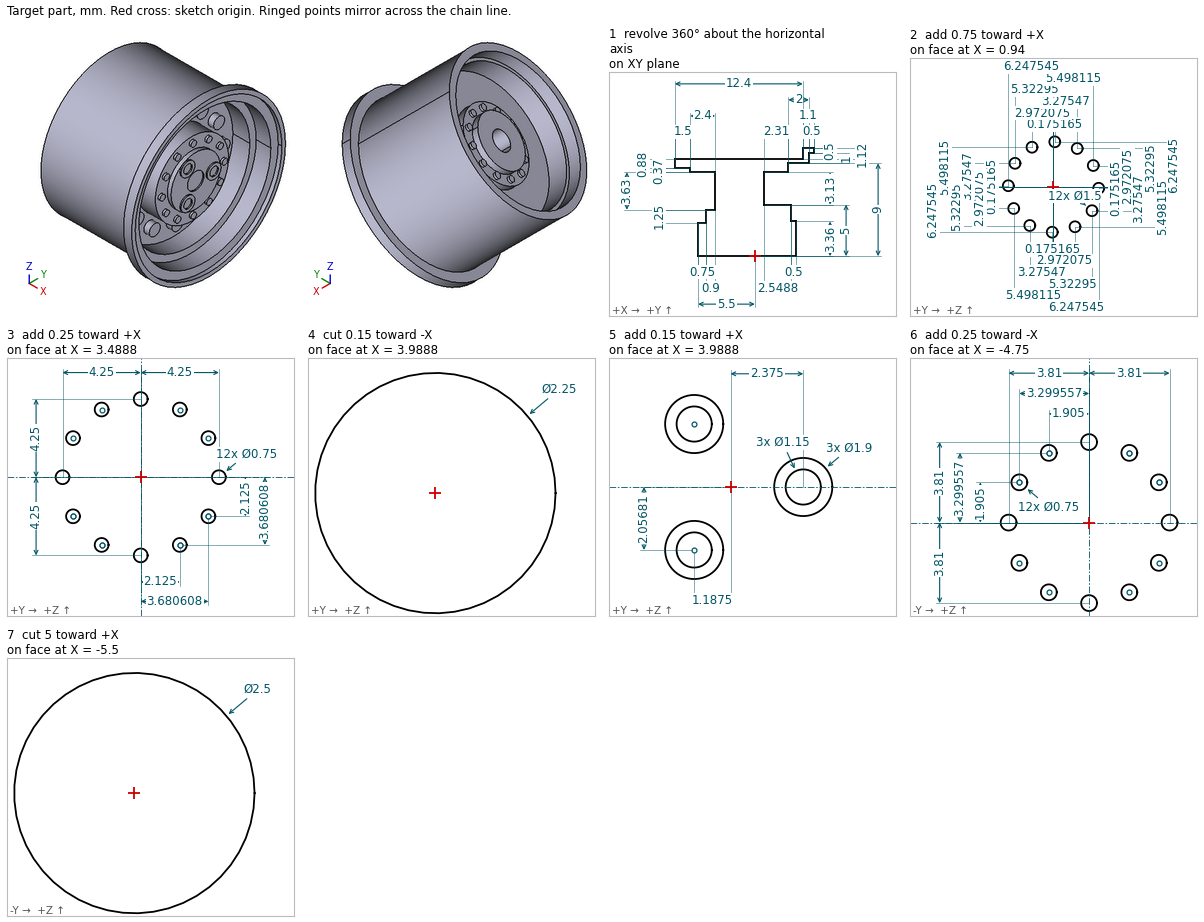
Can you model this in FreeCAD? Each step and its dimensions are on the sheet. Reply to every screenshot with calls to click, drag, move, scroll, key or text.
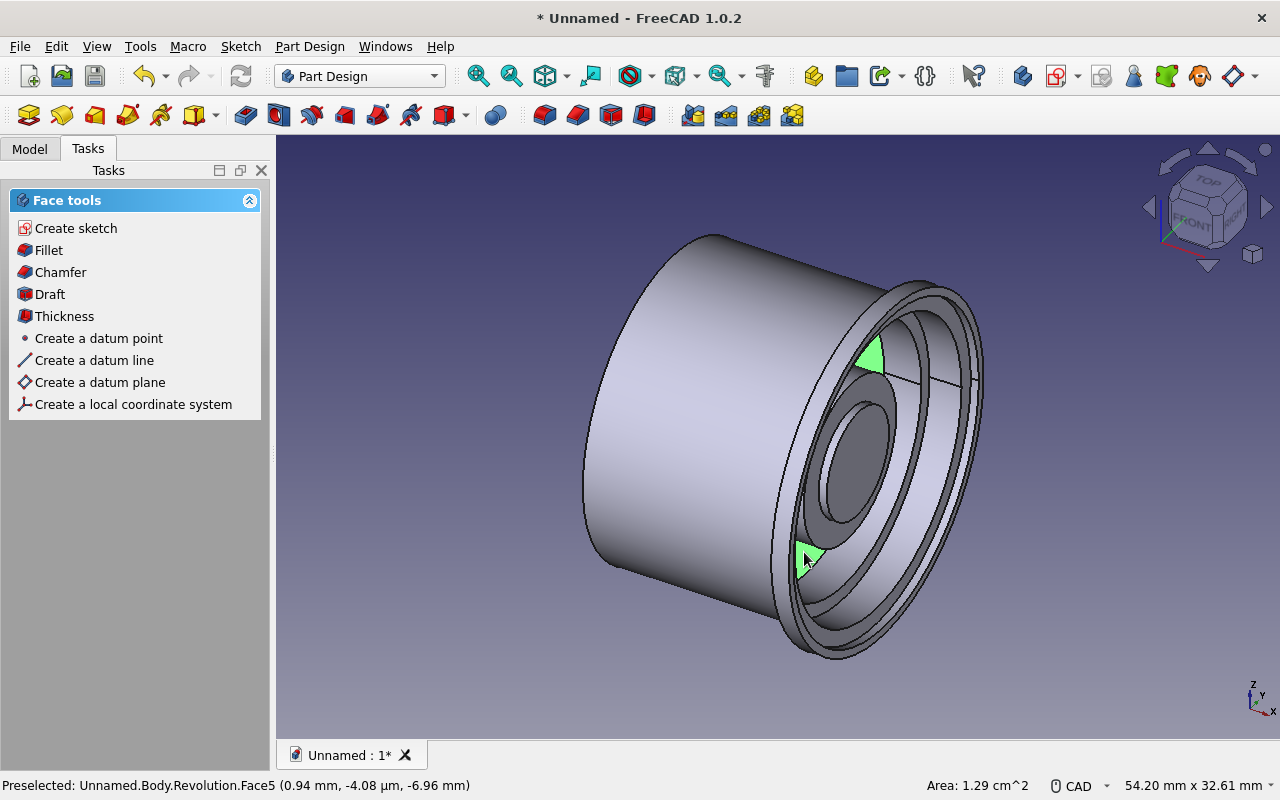
click(1056, 76)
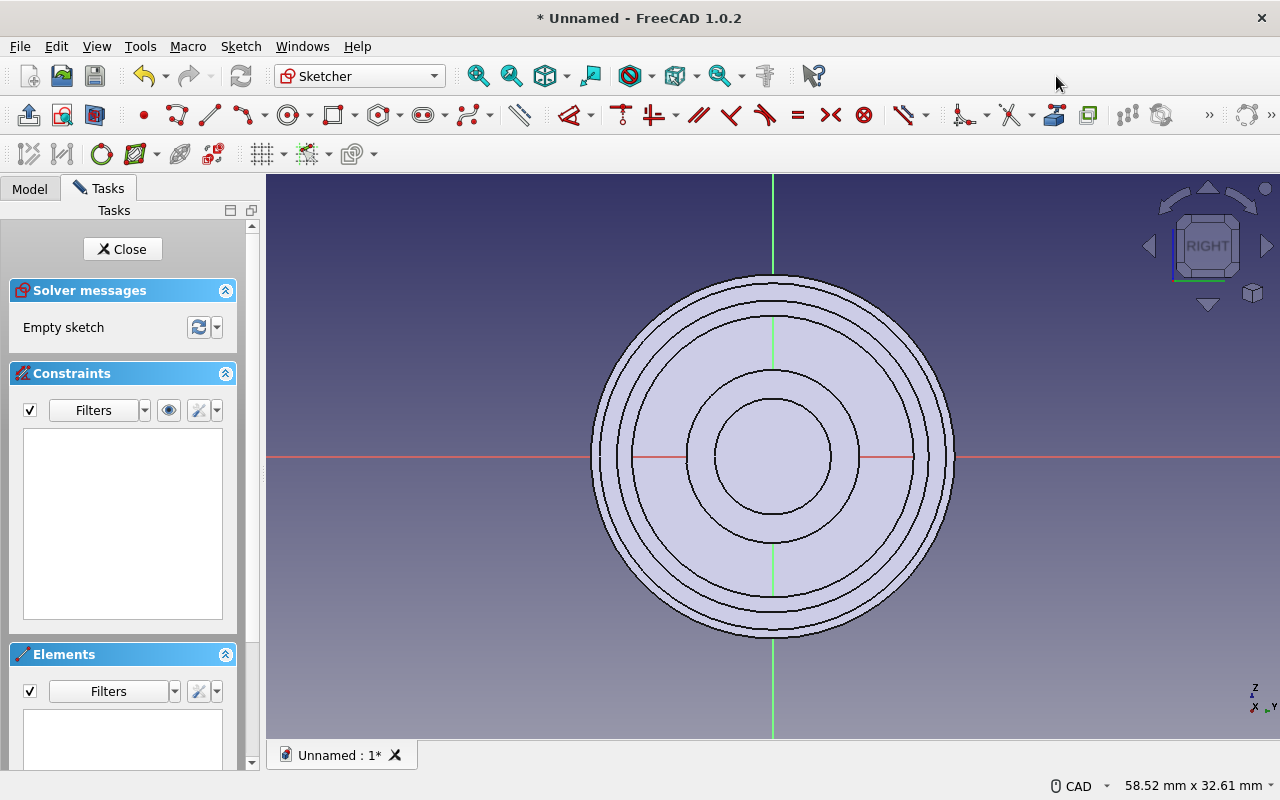
click(95, 116)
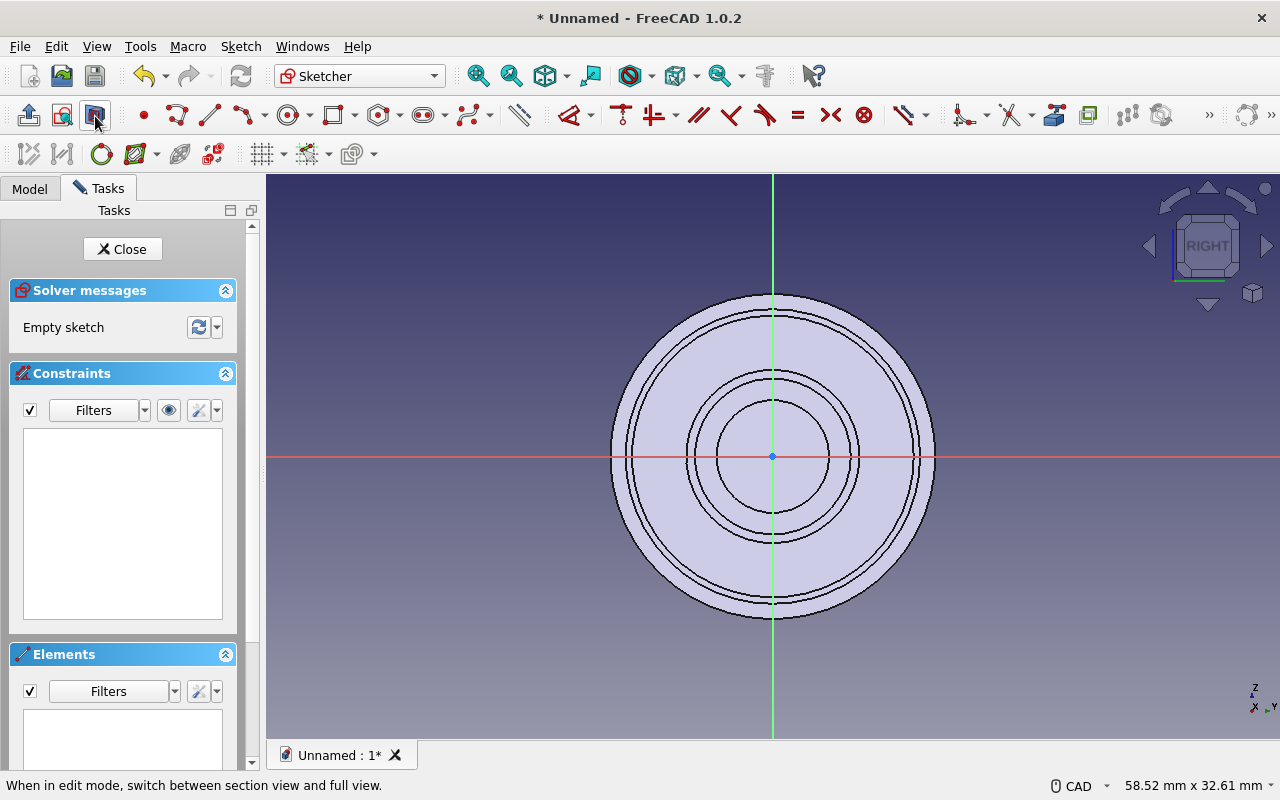
scroll(912, 456, up, 2)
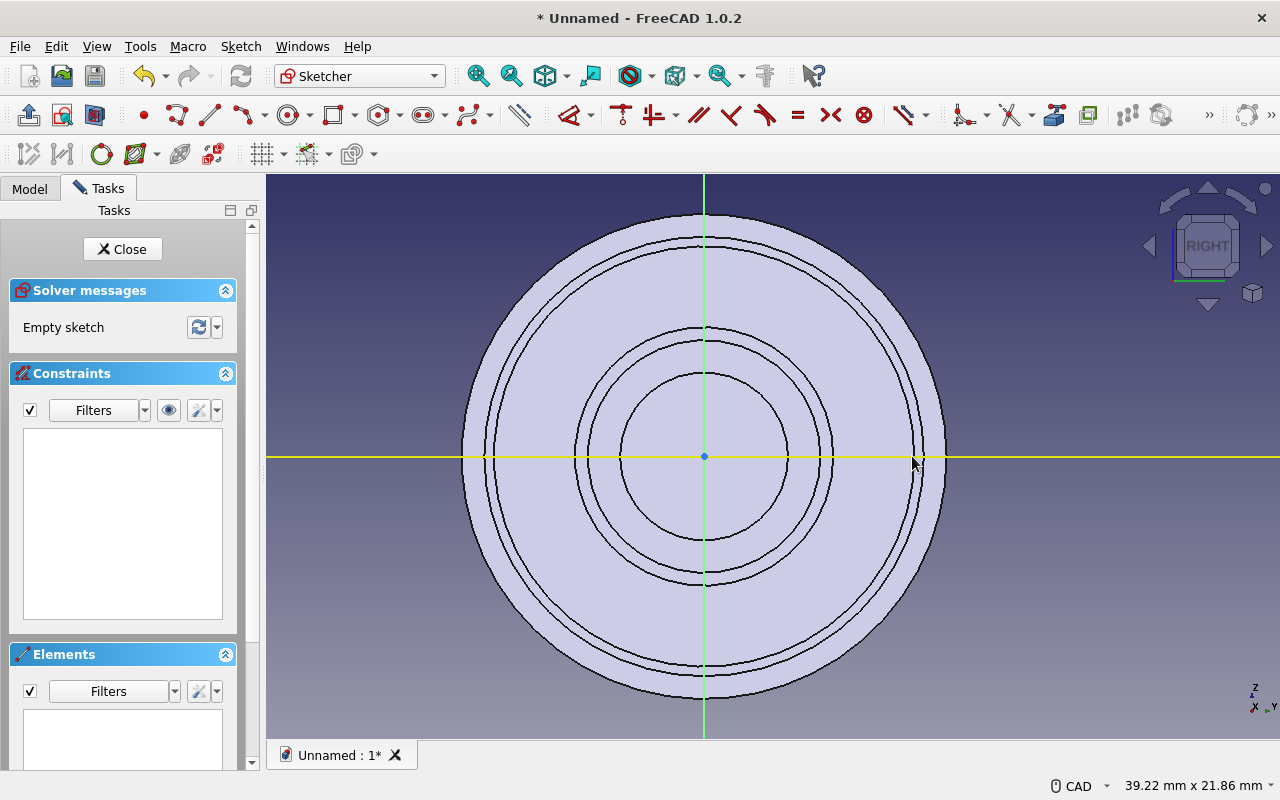
click(288, 116)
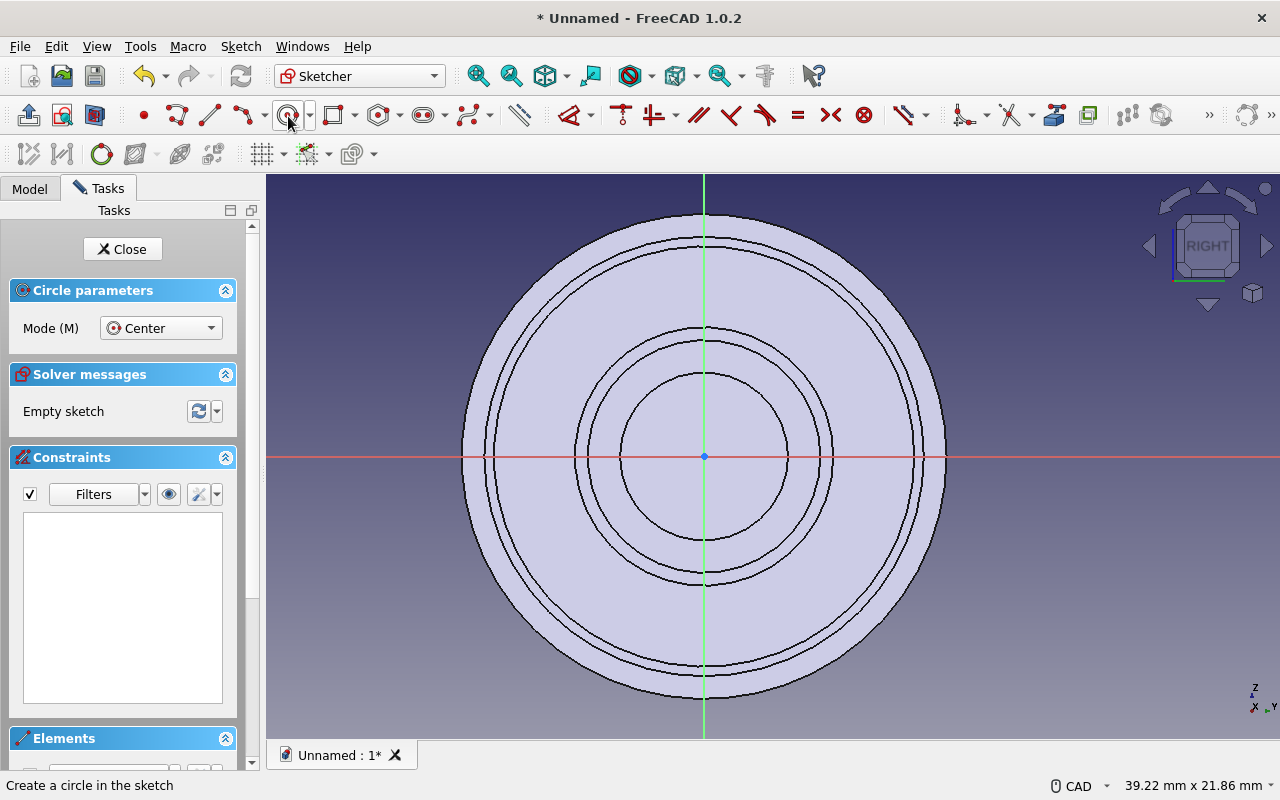
scroll(866, 461, up, 7)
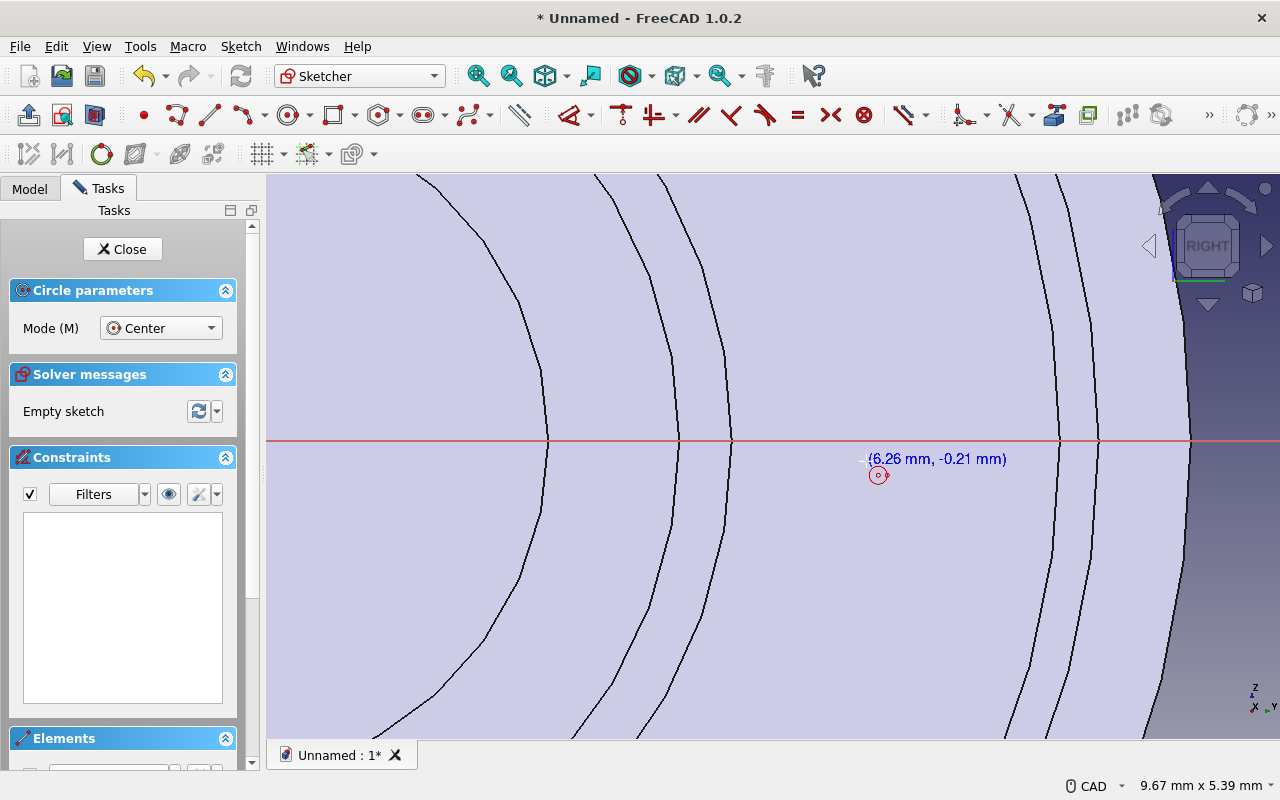
click(863, 460)
move(918, 404)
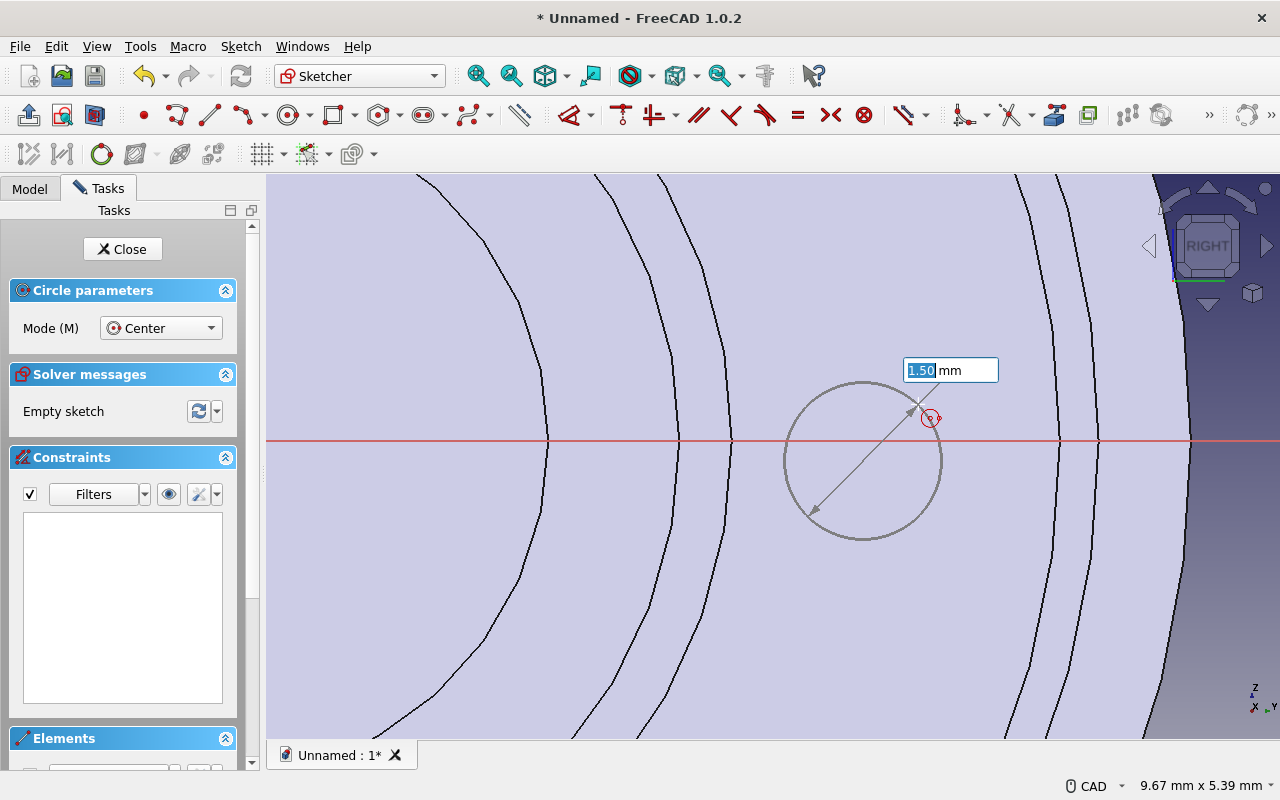
text(1.5)
key(Return)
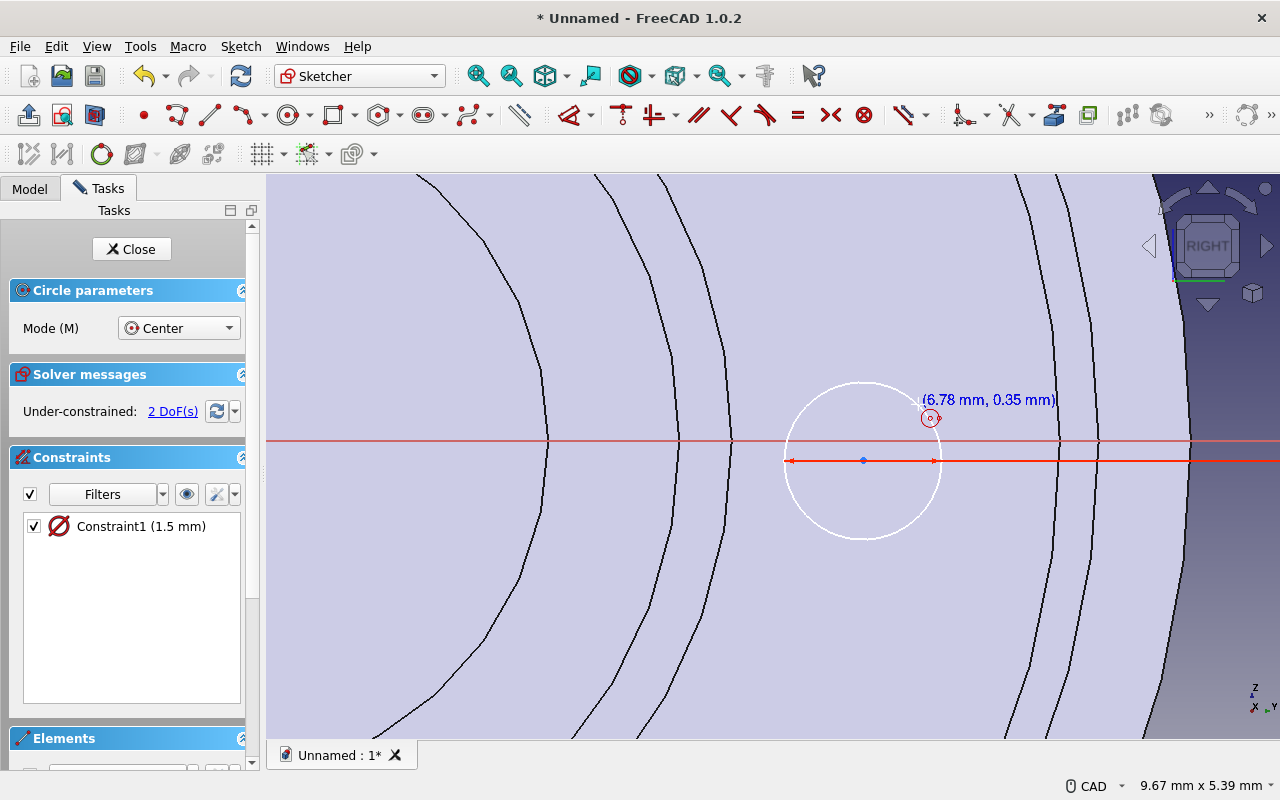
scroll(867, 462, down, 7)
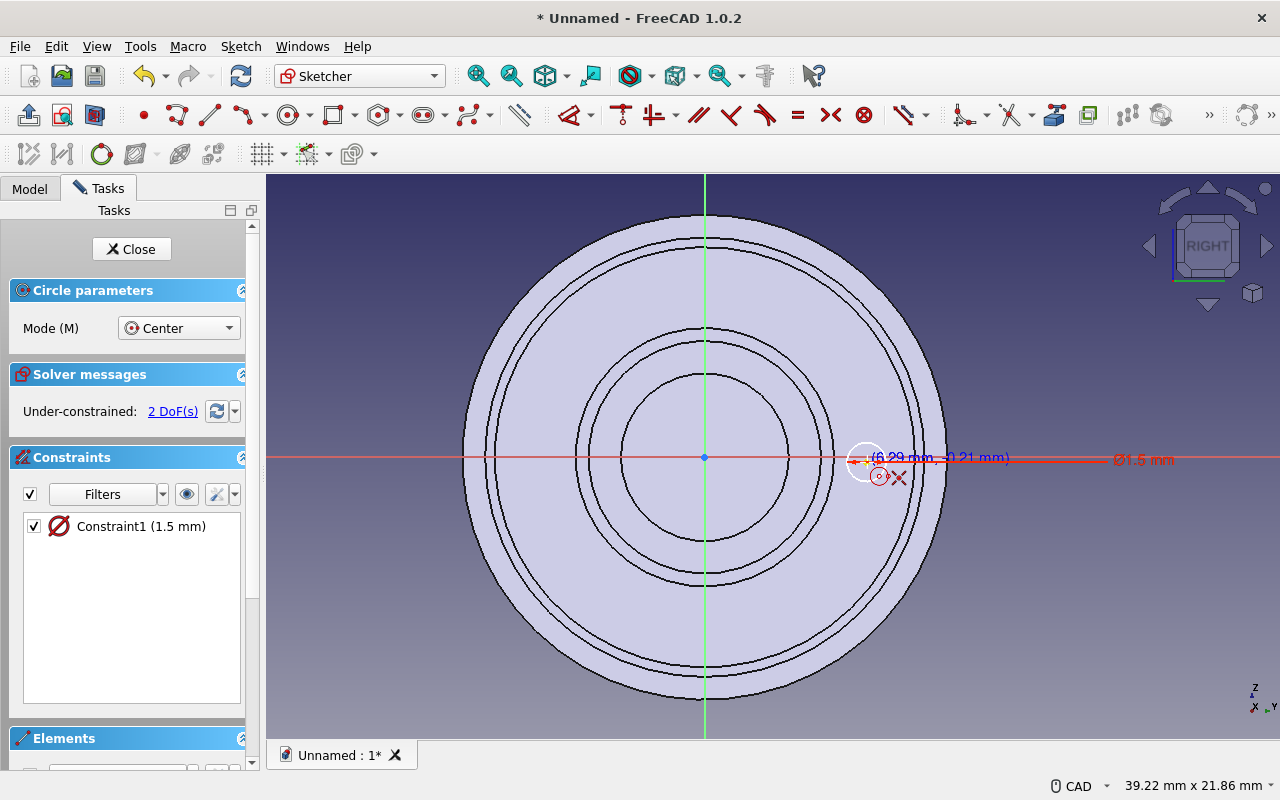
click(842, 542)
move(856, 528)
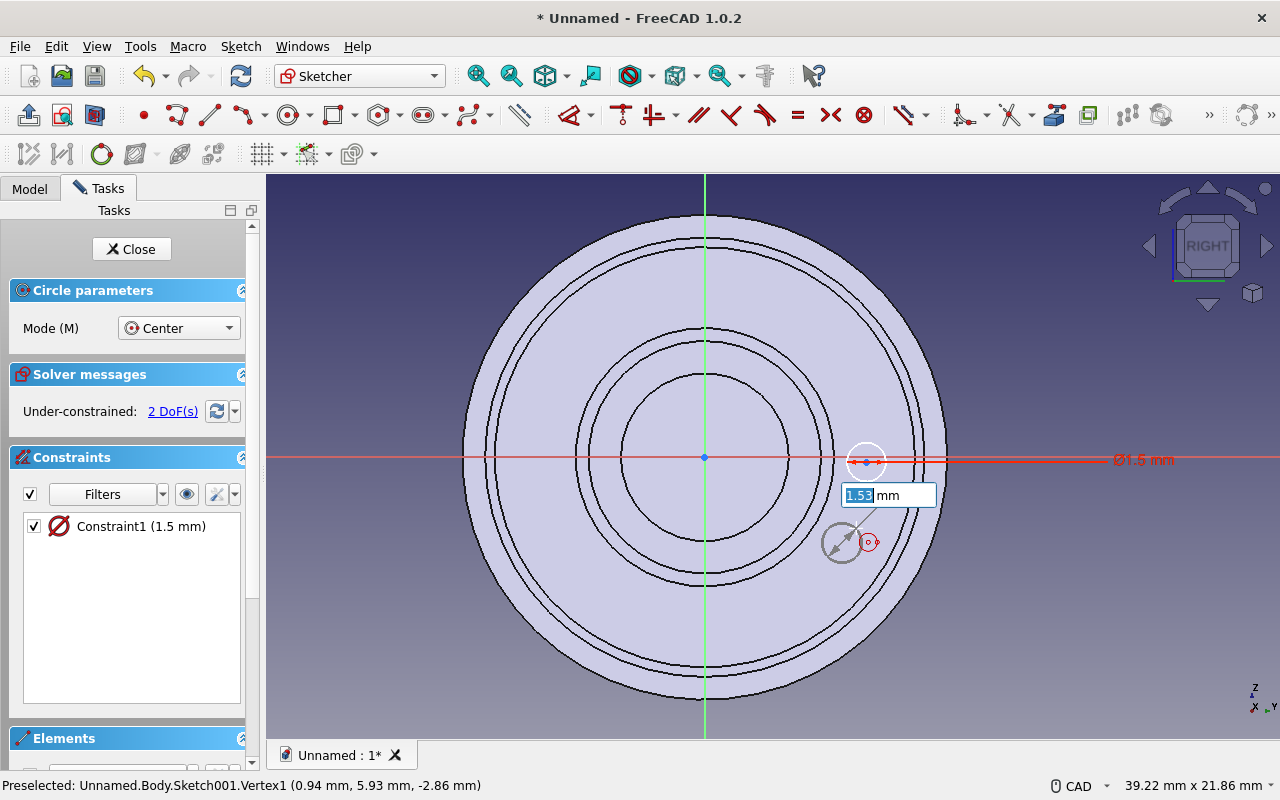
text(1.5)
key(Return)